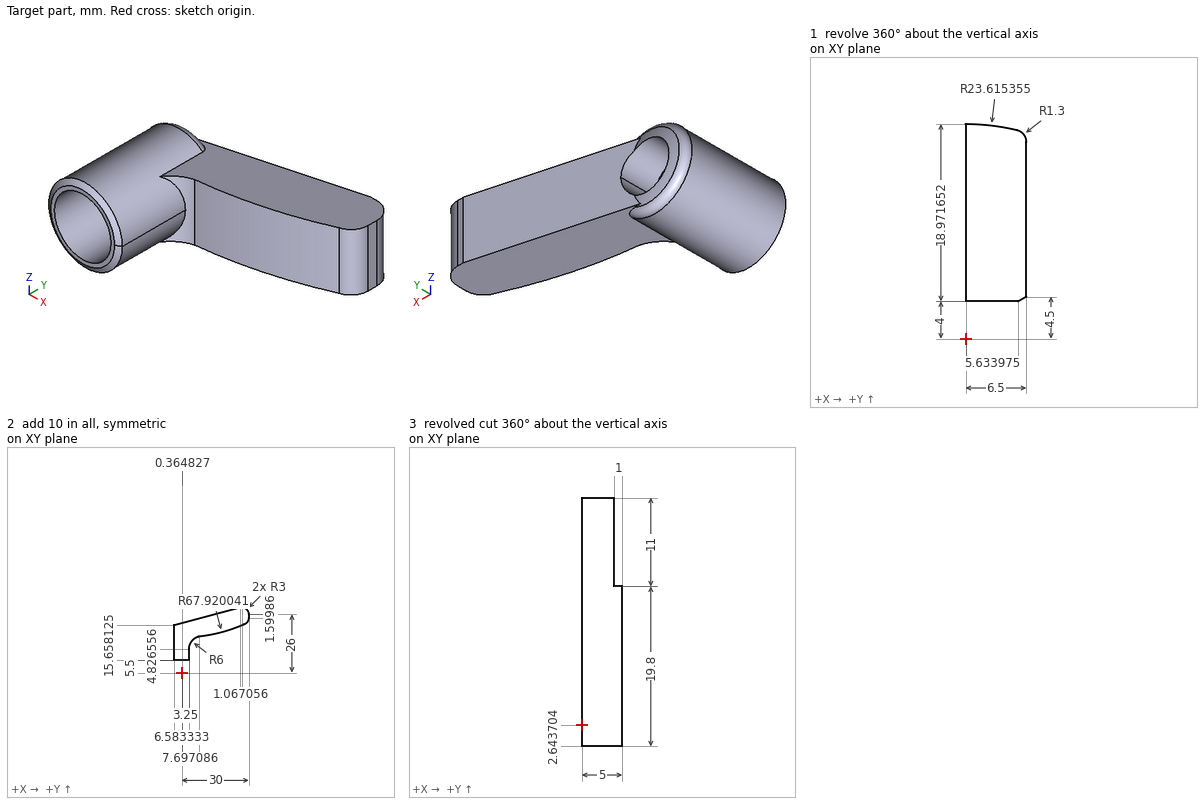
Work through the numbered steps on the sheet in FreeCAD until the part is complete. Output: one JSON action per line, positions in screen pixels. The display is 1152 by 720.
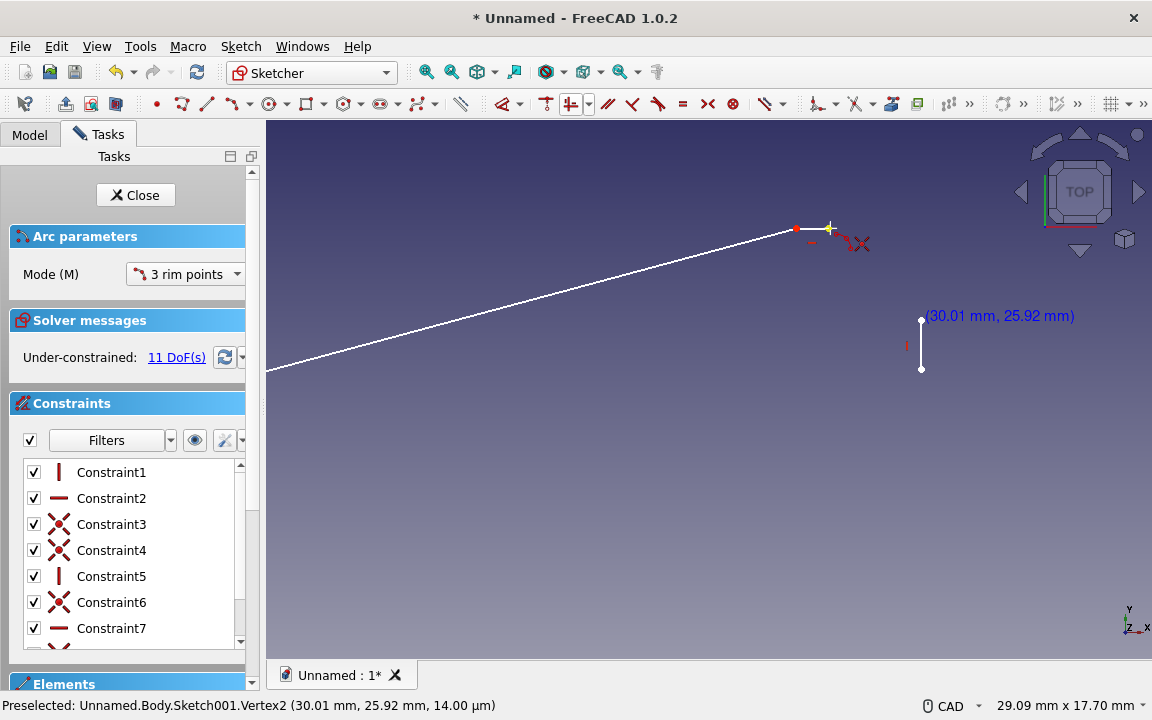
{"action": "left_click", "coordinate": [829, 229]}
{"action": "left_click", "coordinate": [894, 254]}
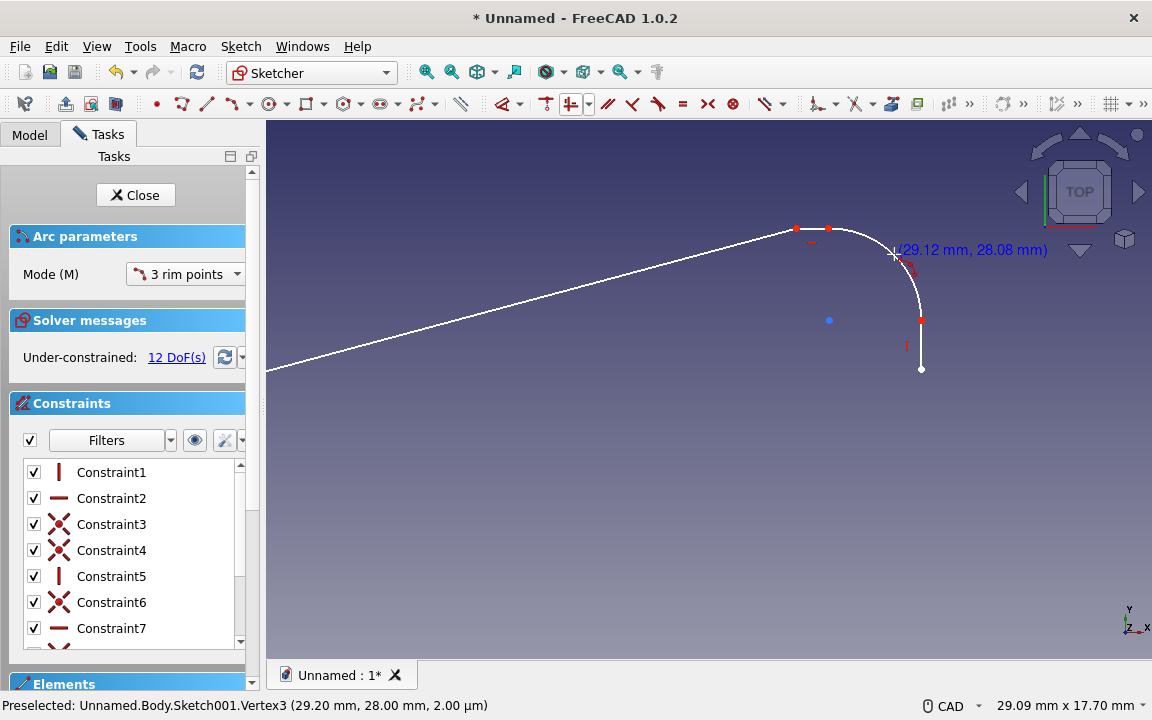
{"action": "scroll", "coordinate": [773, 227], "scroll_direction": "down", "scroll_amount": 5}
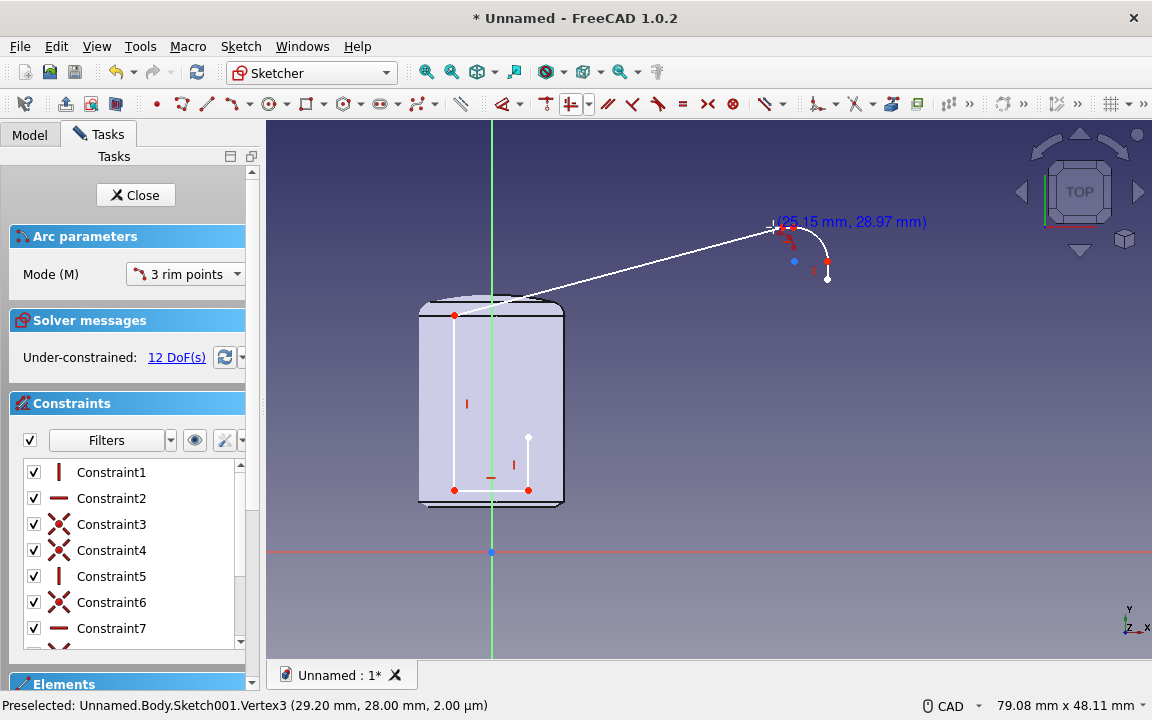
{"action": "left_click", "coordinate": [528, 437]}
{"action": "left_click", "coordinate": [578, 371]}
{"action": "left_click", "coordinate": [542, 395]}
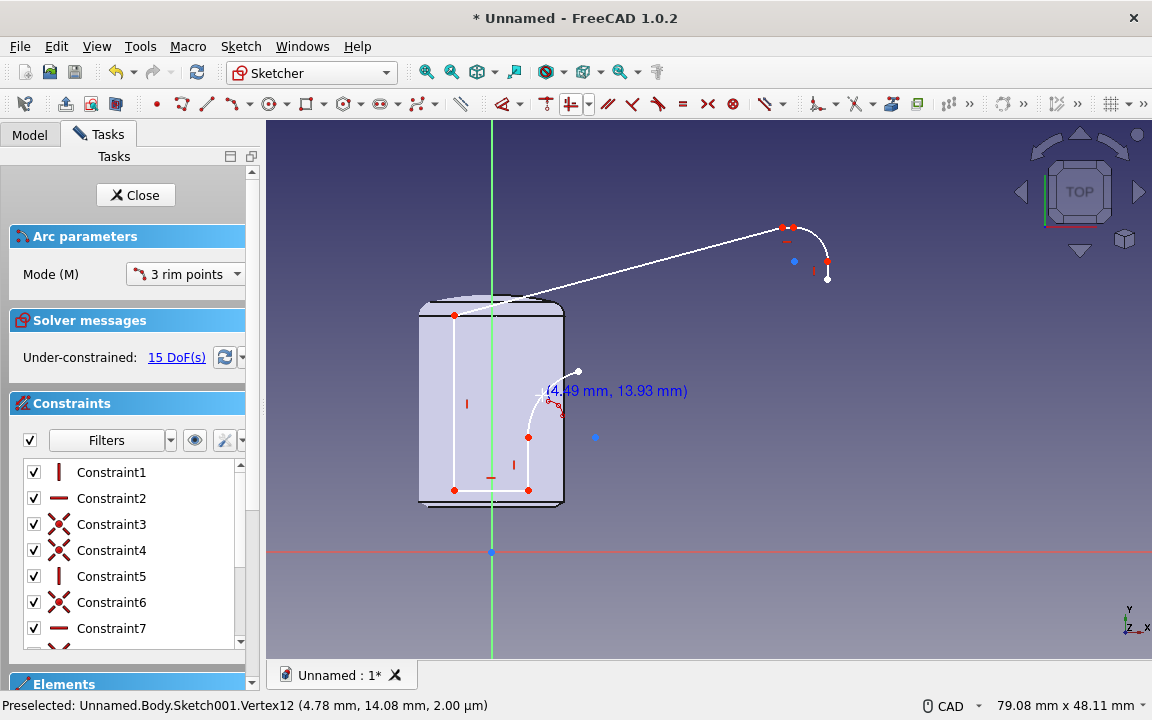
{"action": "left_click", "coordinate": [578, 372]}
{"action": "left_click", "coordinate": [803, 311]}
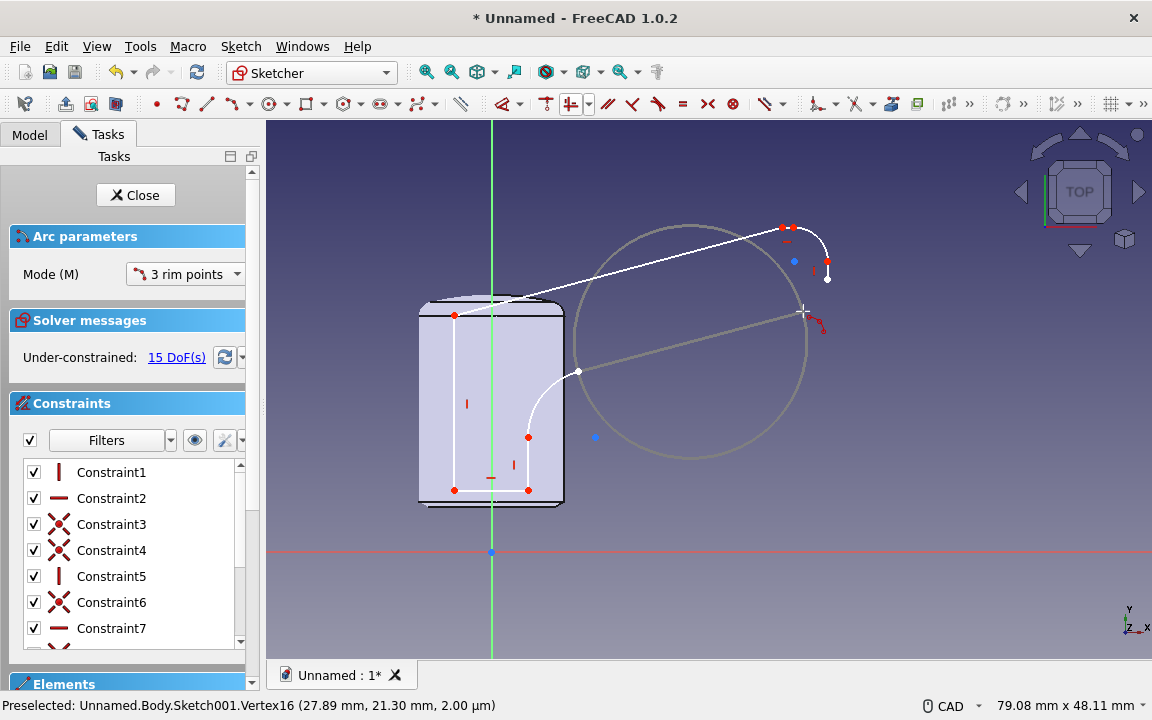
{"action": "scroll", "coordinate": [693, 350], "scroll_direction": "up", "scroll_amount": 3}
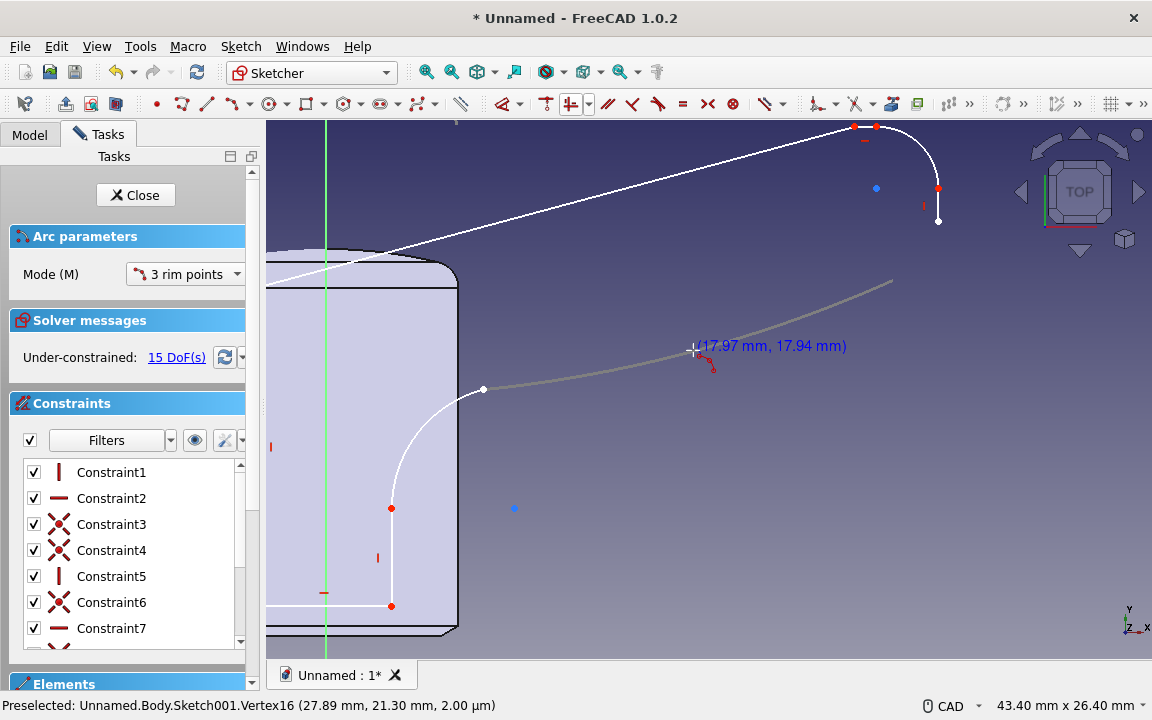
{"action": "left_click", "coordinate": [692, 350]}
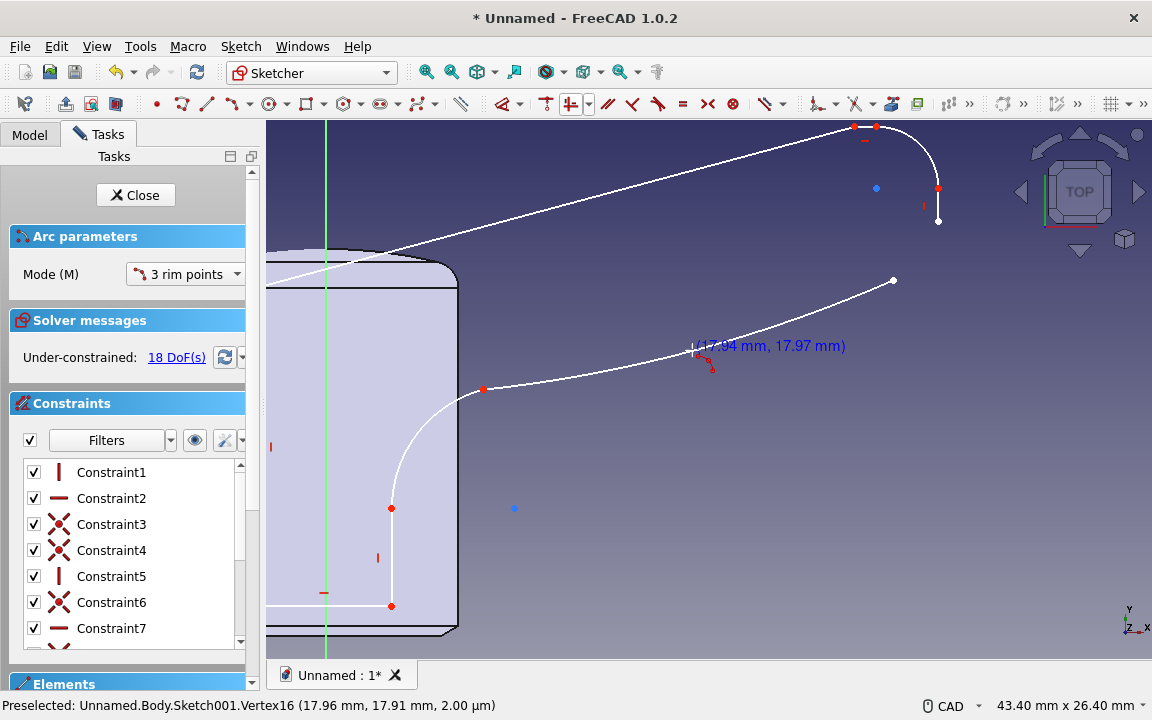
{"action": "left_click", "coordinate": [893, 280]}
{"action": "left_click", "coordinate": [938, 222]}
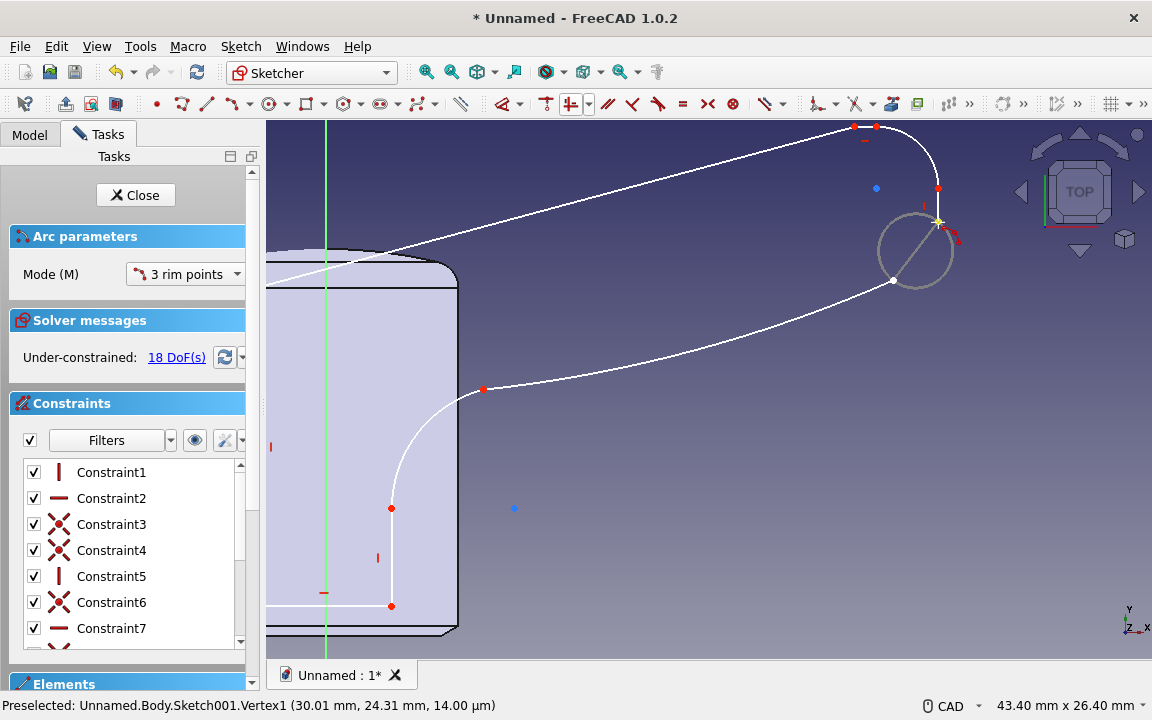
{"action": "scroll", "coordinate": [925, 257], "scroll_direction": "up", "scroll_amount": 2}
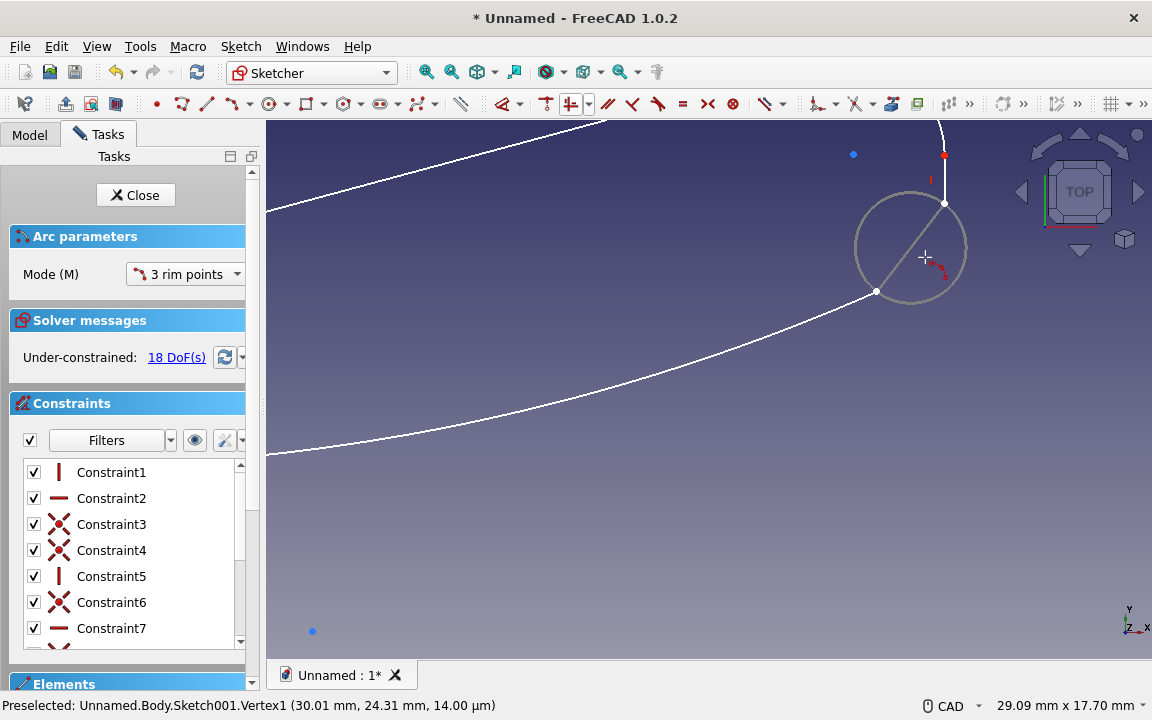
{"action": "left_click", "coordinate": [925, 257]}
{"action": "key", "text": "Escape"}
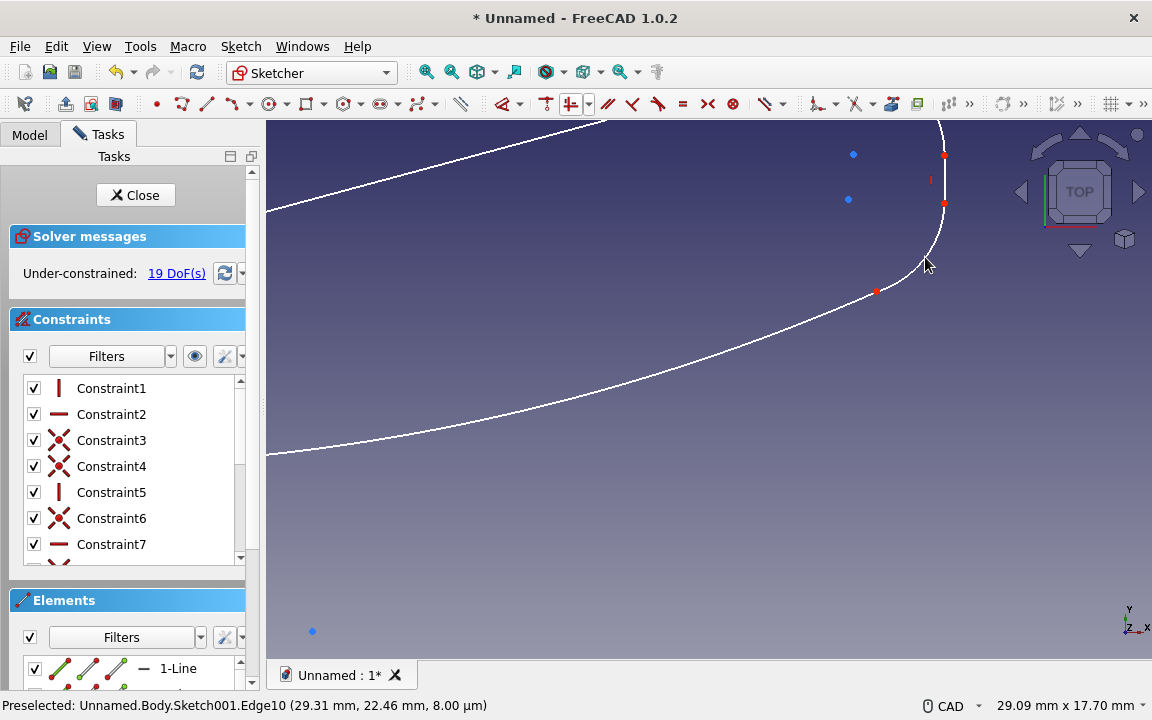
{"action": "left_click", "coordinate": [945, 189]}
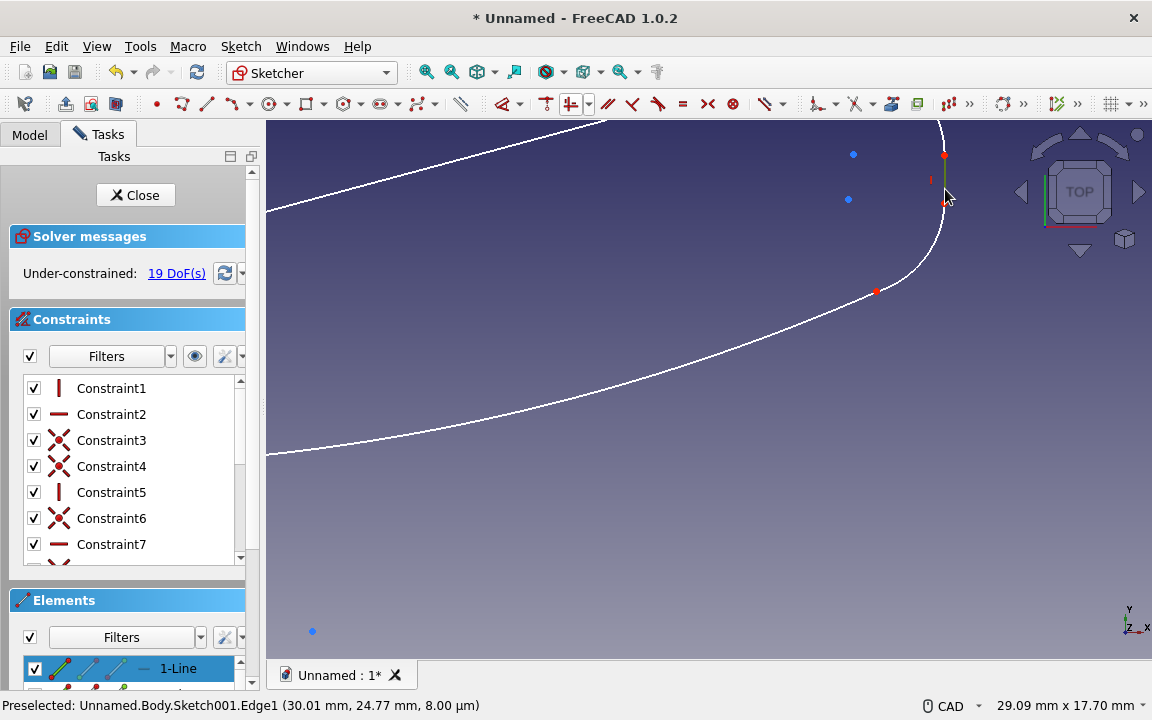
{"action": "scroll", "coordinate": [759, 324], "scroll_direction": "down", "scroll_amount": 5}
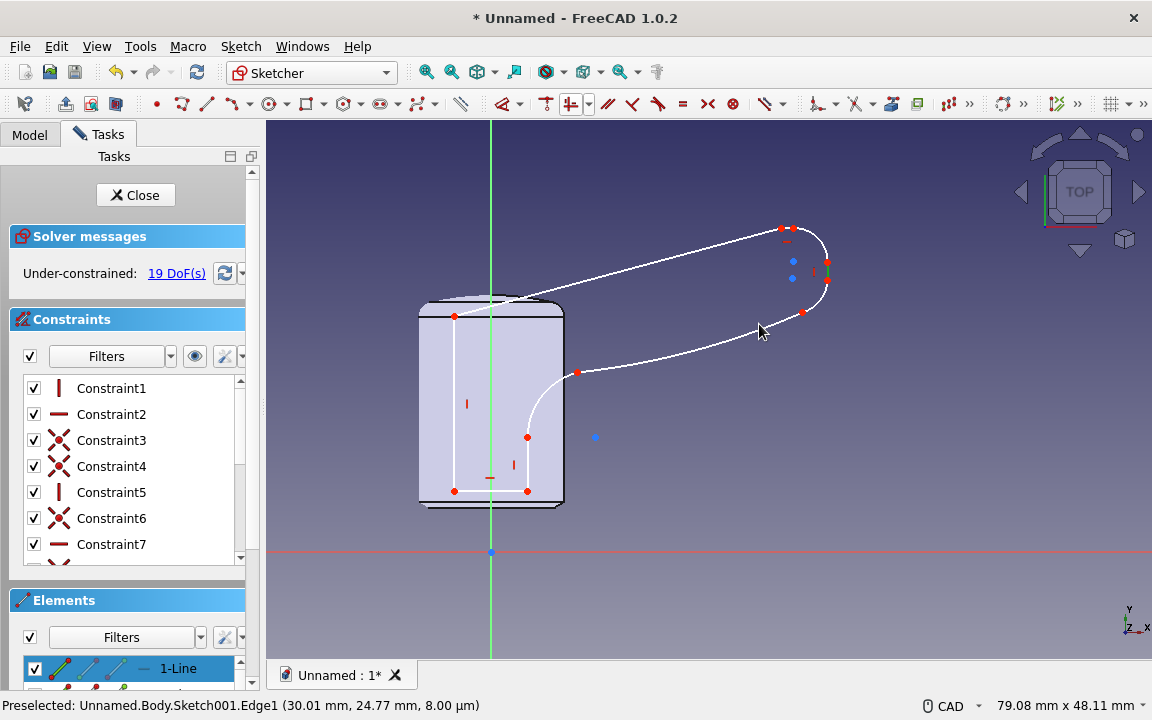
{"action": "left_click", "coordinate": [824, 247]}